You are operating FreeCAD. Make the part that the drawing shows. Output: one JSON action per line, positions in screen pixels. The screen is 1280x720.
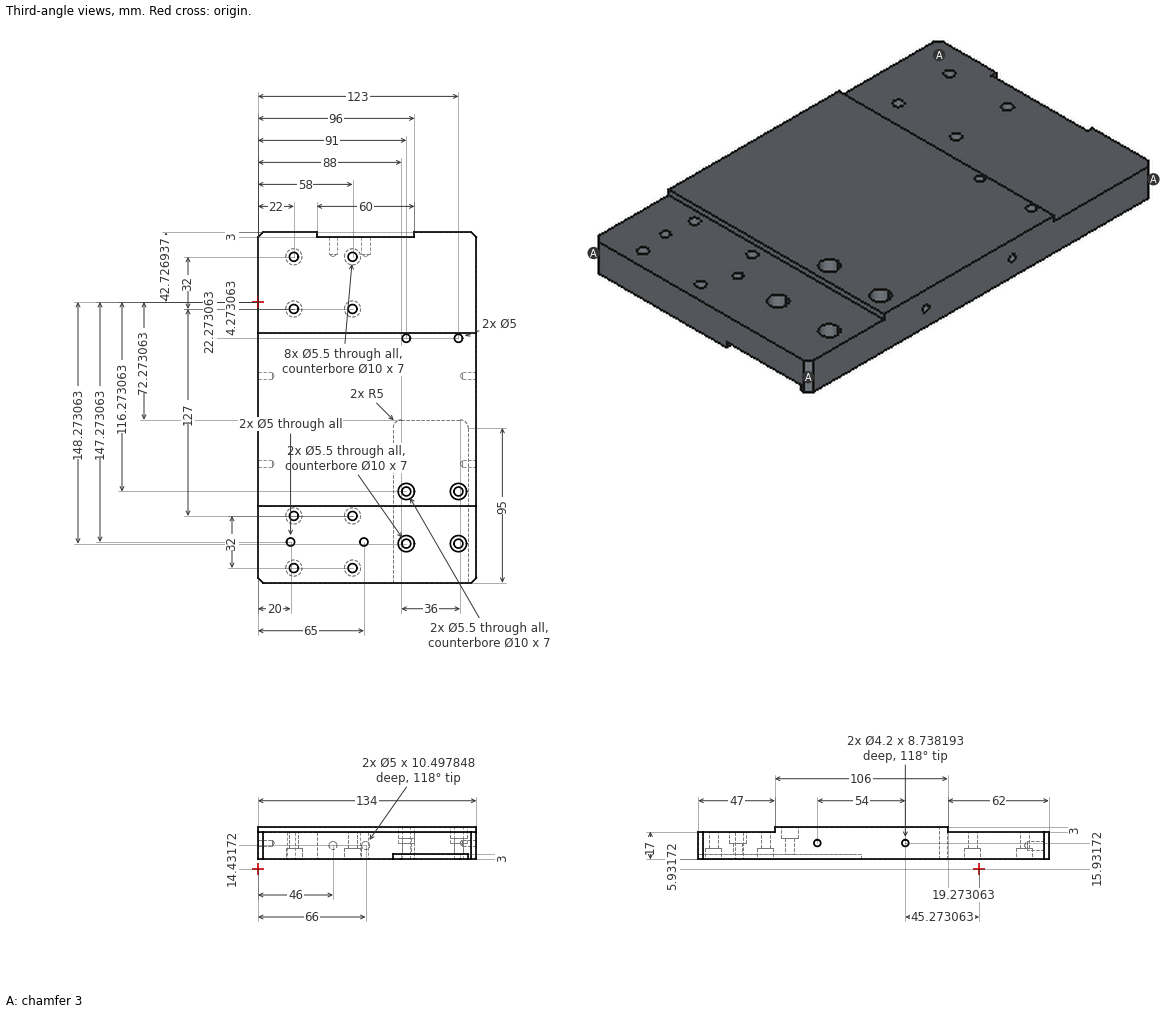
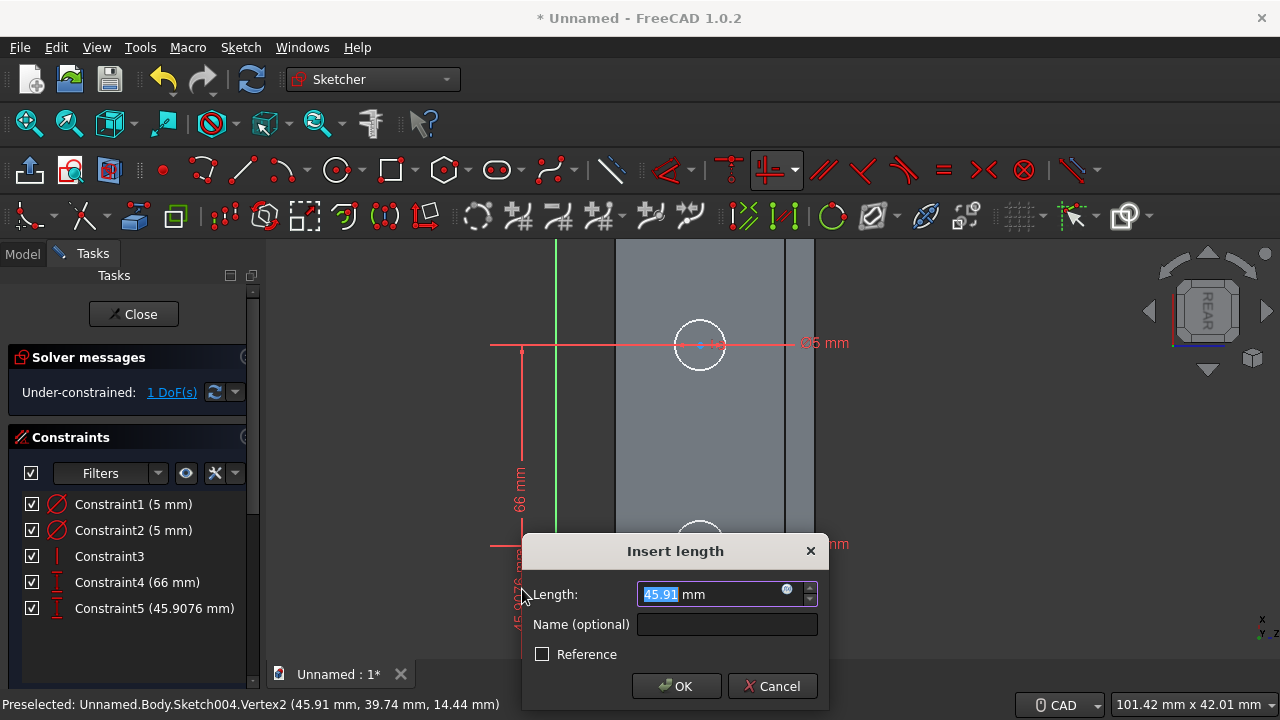
{"action": "type", "text": "46"}
{"action": "key", "text": "Return"}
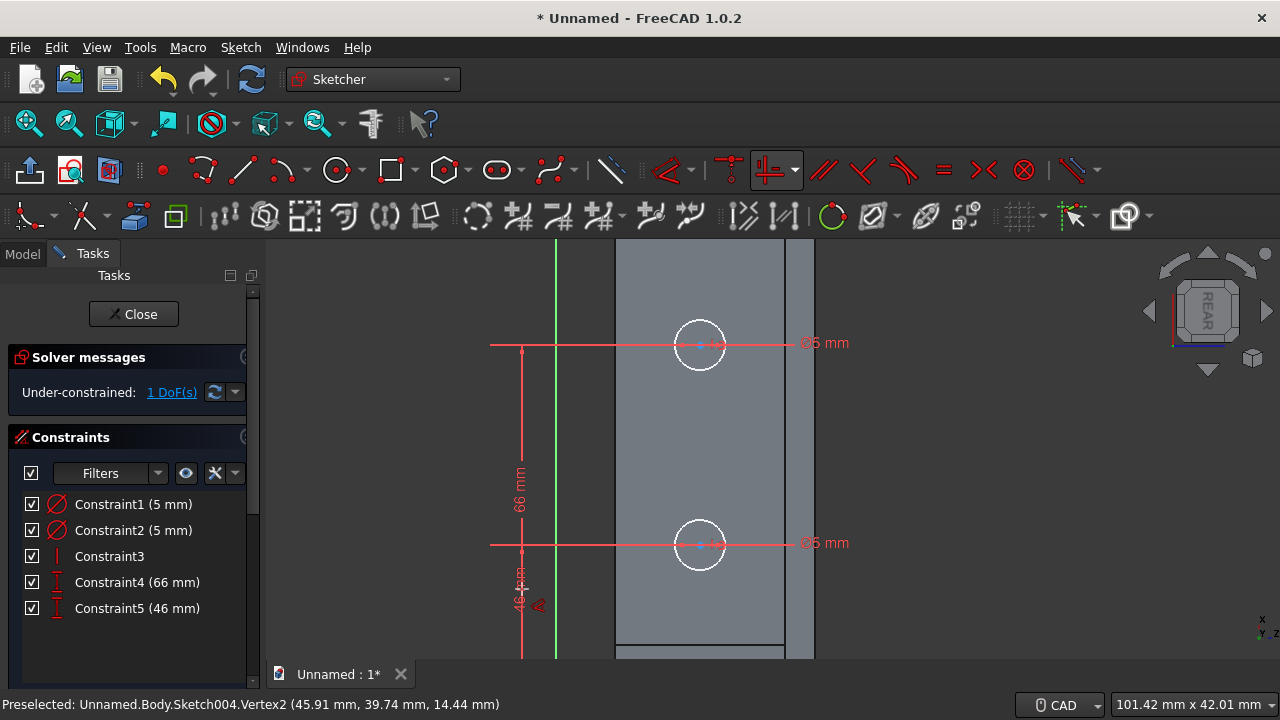
{"action": "left_click", "coordinate": [700, 345]}
{"action": "left_click", "coordinate": [628, 311]}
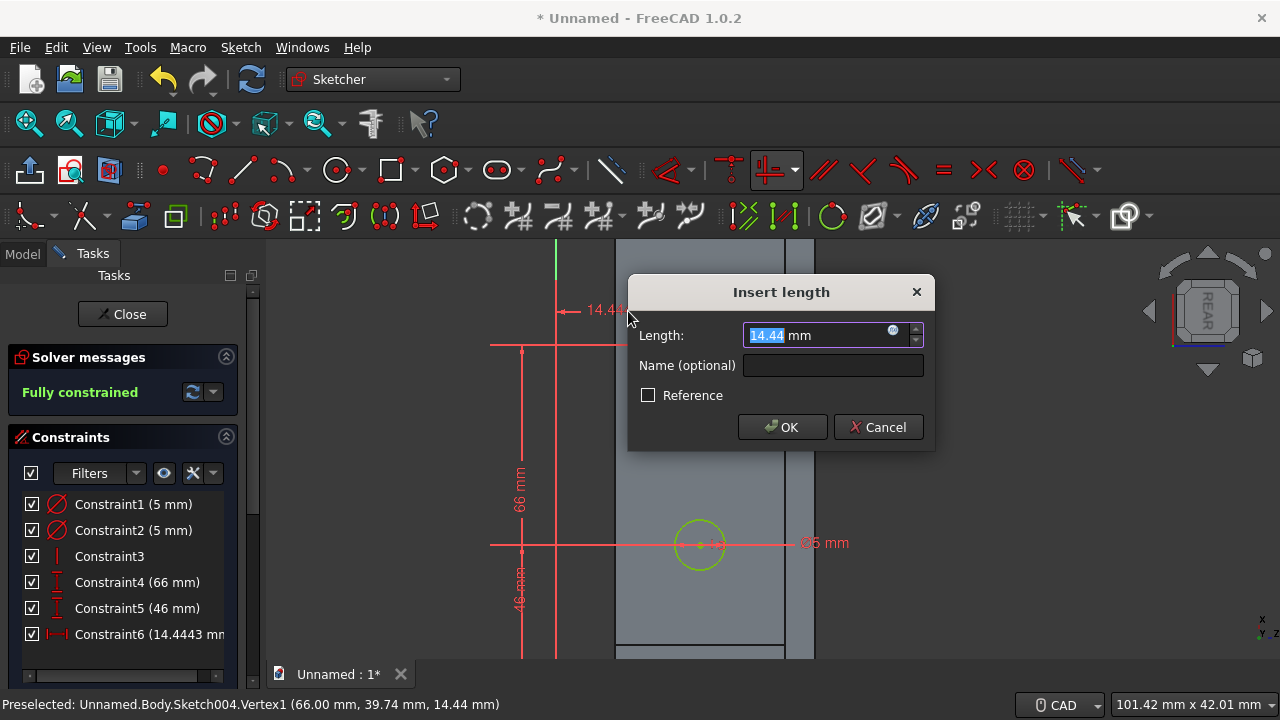
{"action": "type", "text": "14.43172"}
{"action": "key", "text": "Return"}
{"action": "key", "text": "Escape"}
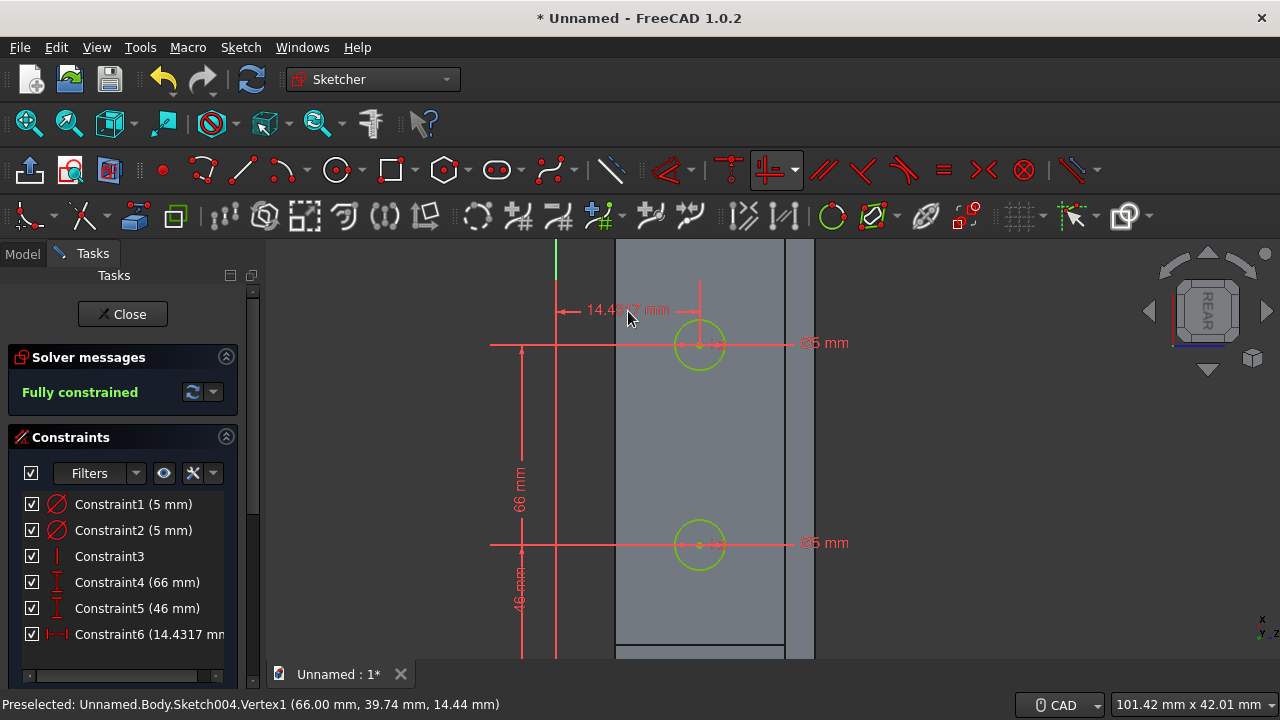
{"action": "left_click", "coordinate": [123, 314]}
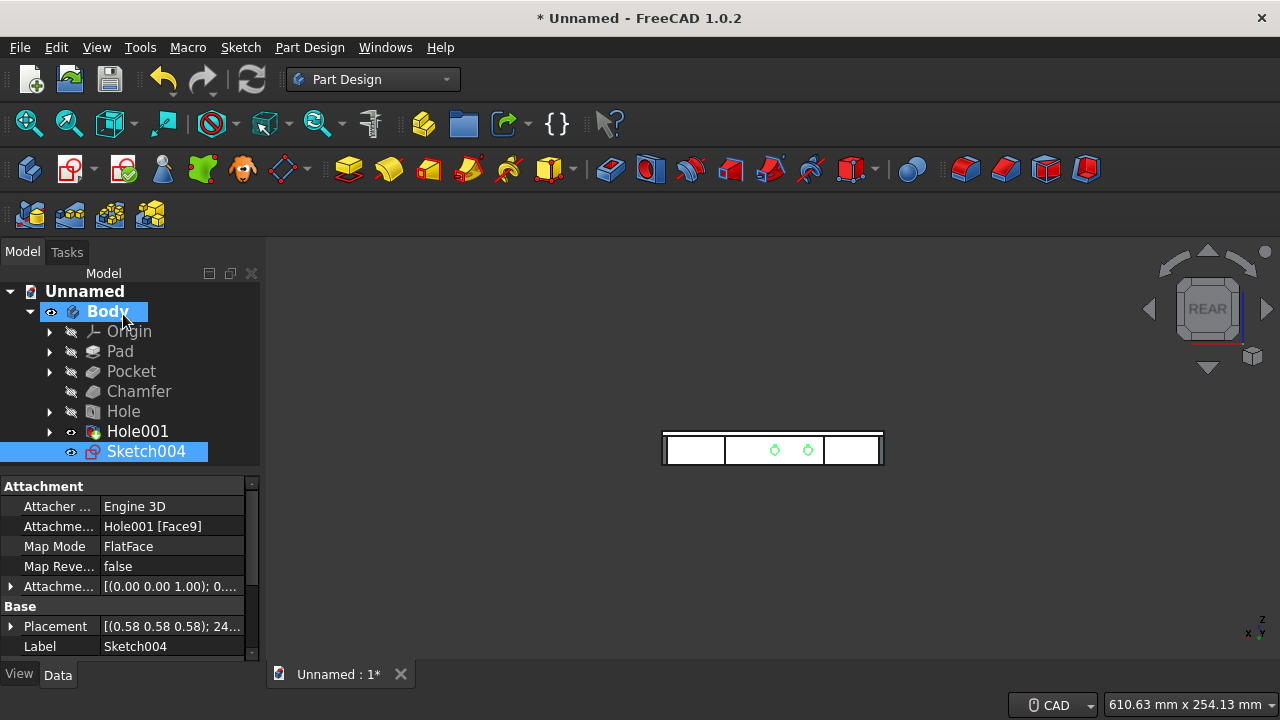
{"action": "left_click", "coordinate": [652, 170]}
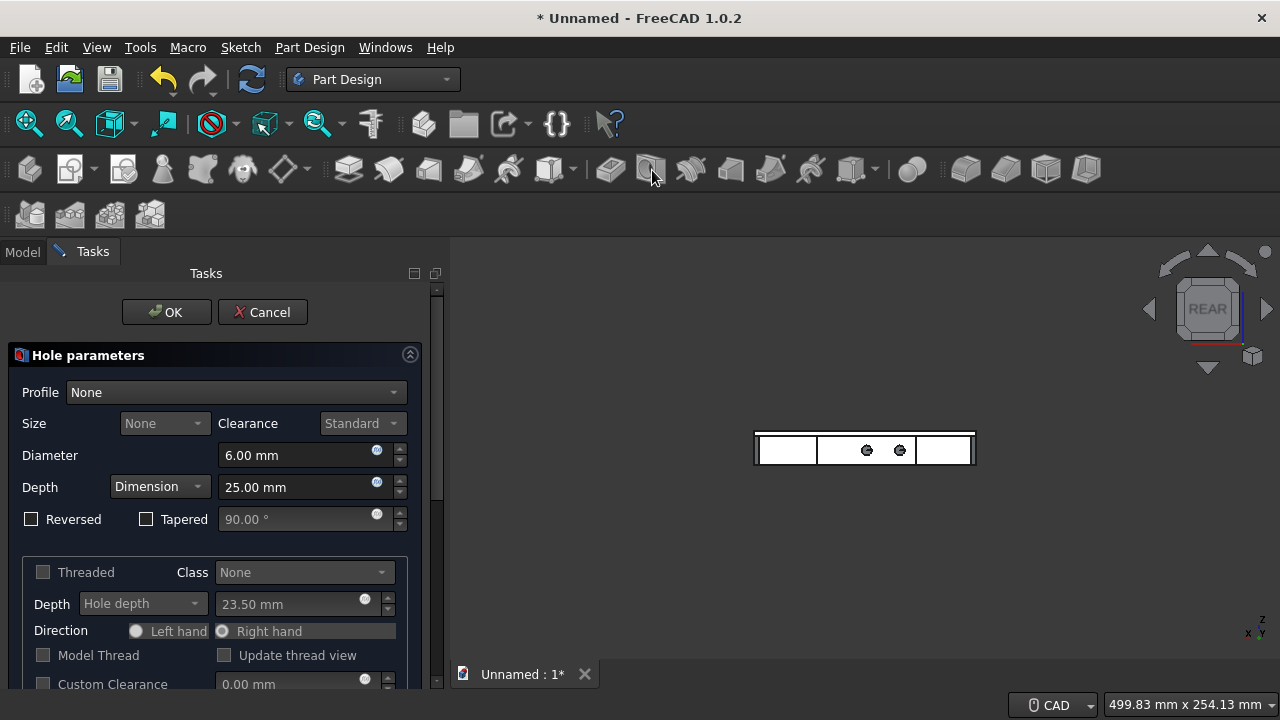
{"action": "triple_click", "coordinate": [305, 455]}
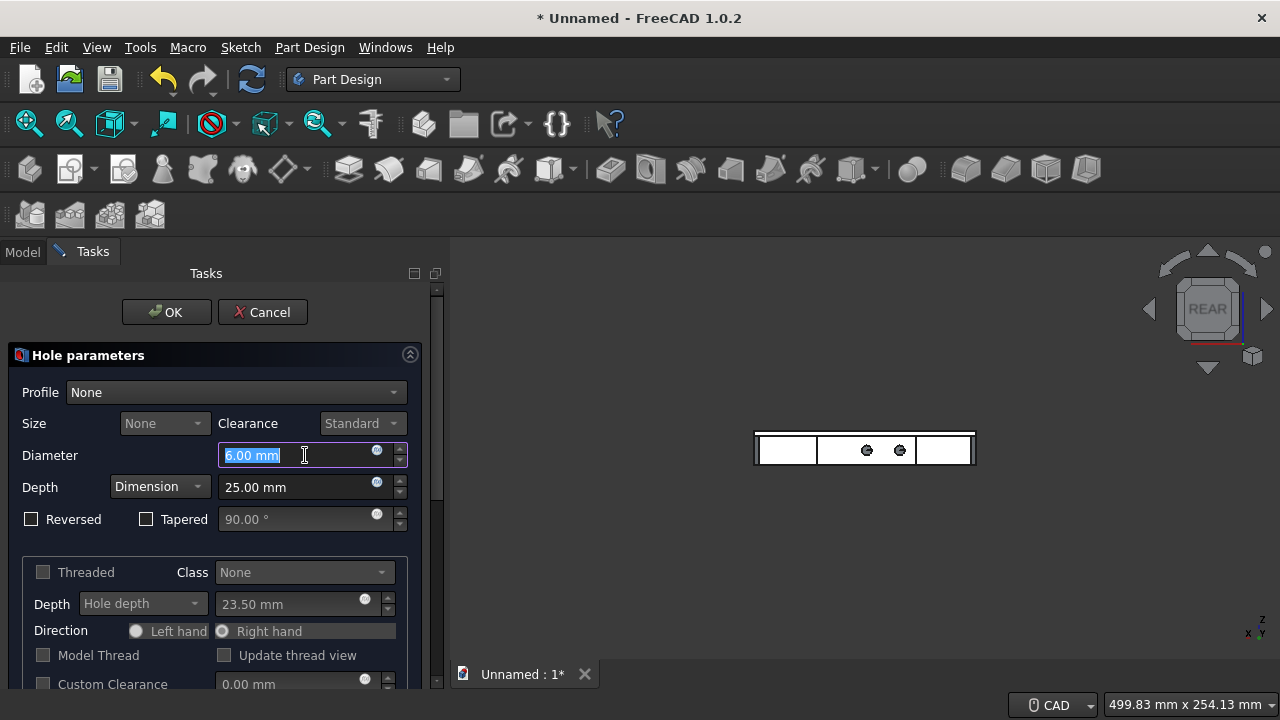
{"action": "type", "text": "5"}
{"action": "key", "text": "Tab"}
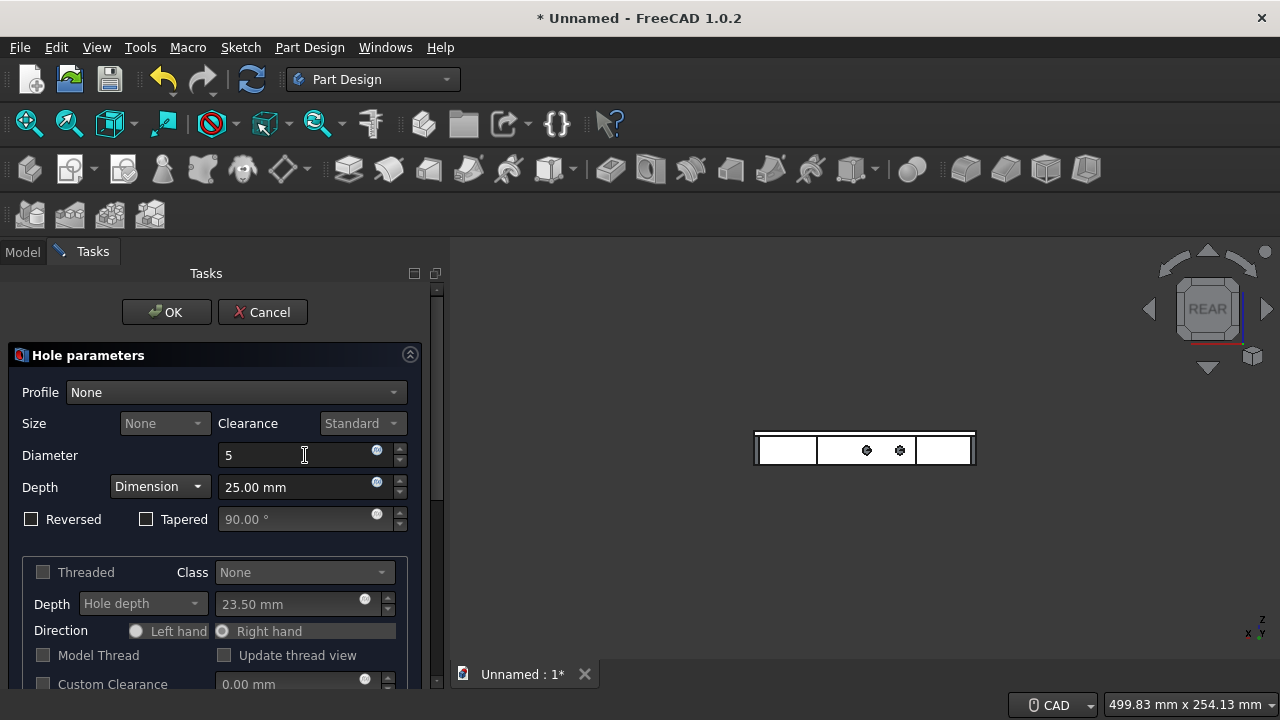
{"action": "triple_click", "coordinate": [305, 487]}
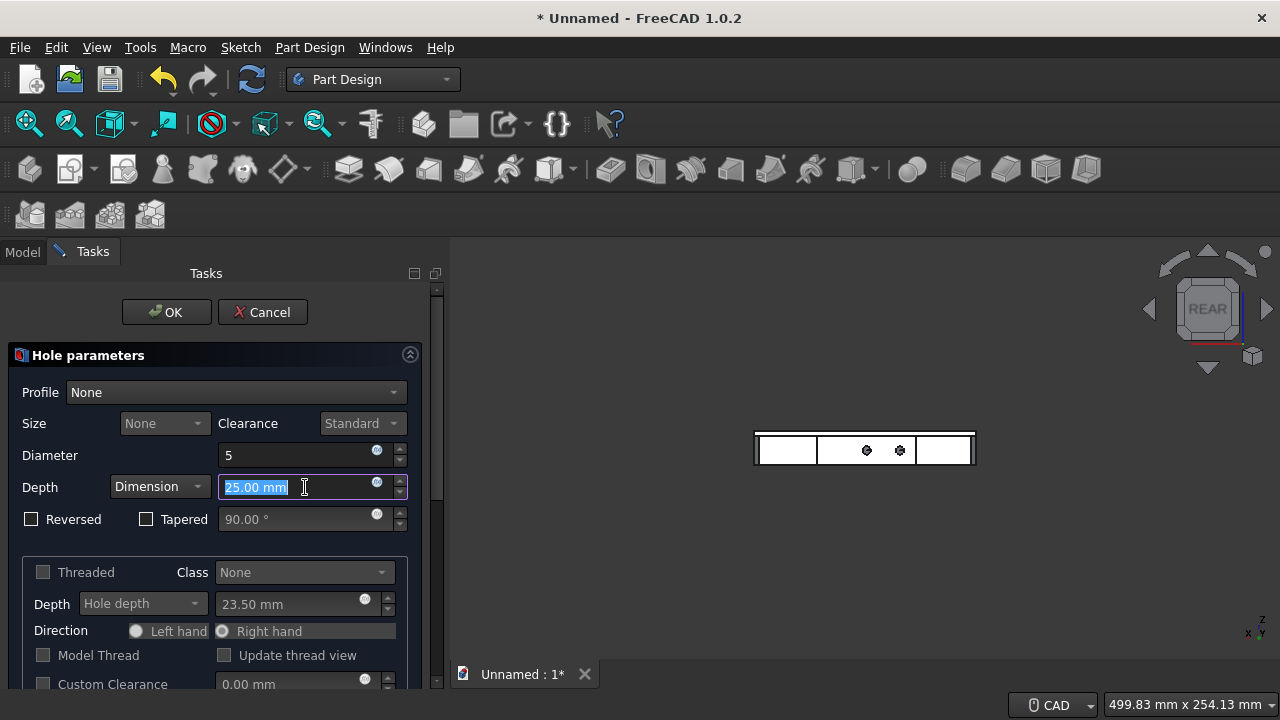
{"action": "type", "text": "10.497848"}
{"action": "key", "text": "Tab"}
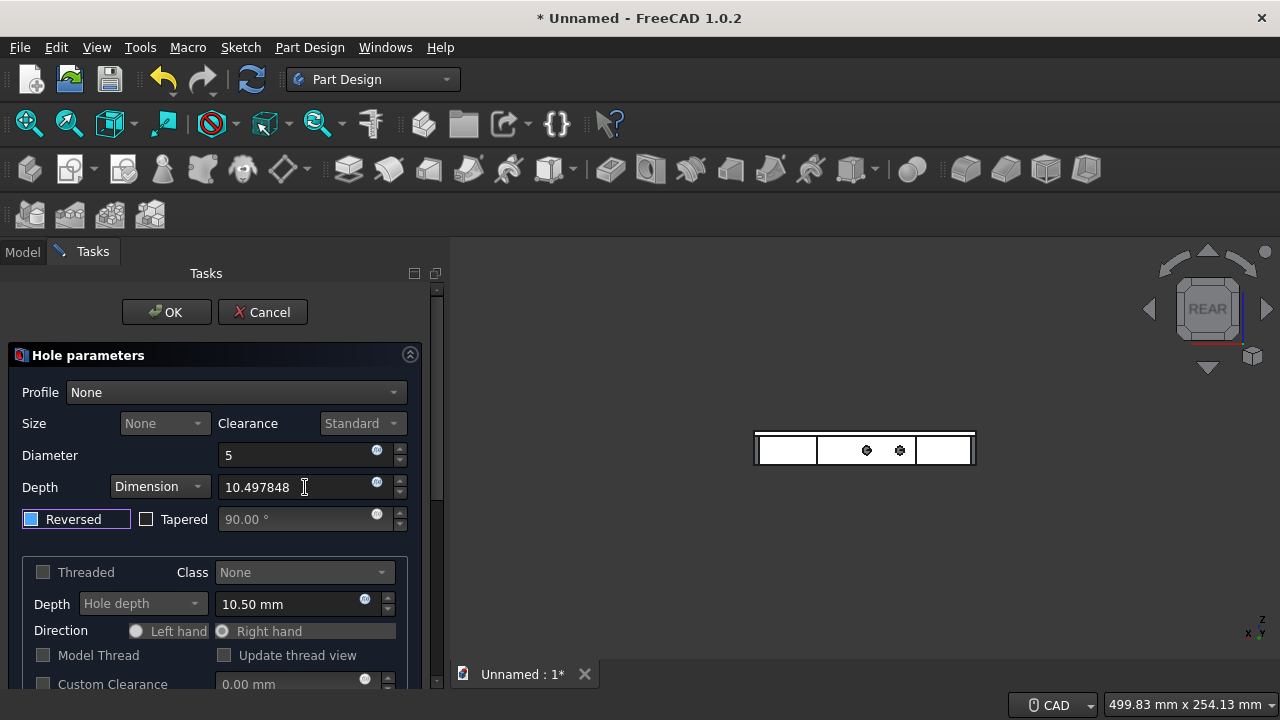
{"action": "left_click", "coordinate": [167, 312]}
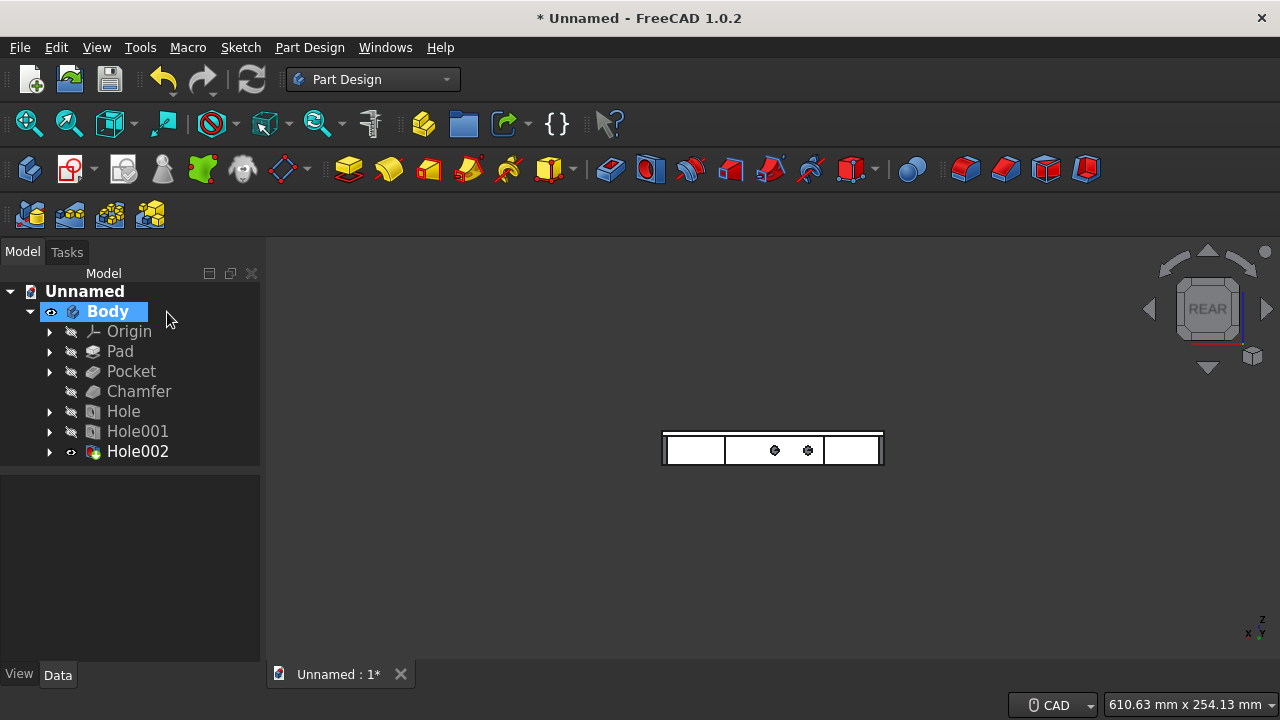
{"action": "left_click", "coordinate": [30, 124]}